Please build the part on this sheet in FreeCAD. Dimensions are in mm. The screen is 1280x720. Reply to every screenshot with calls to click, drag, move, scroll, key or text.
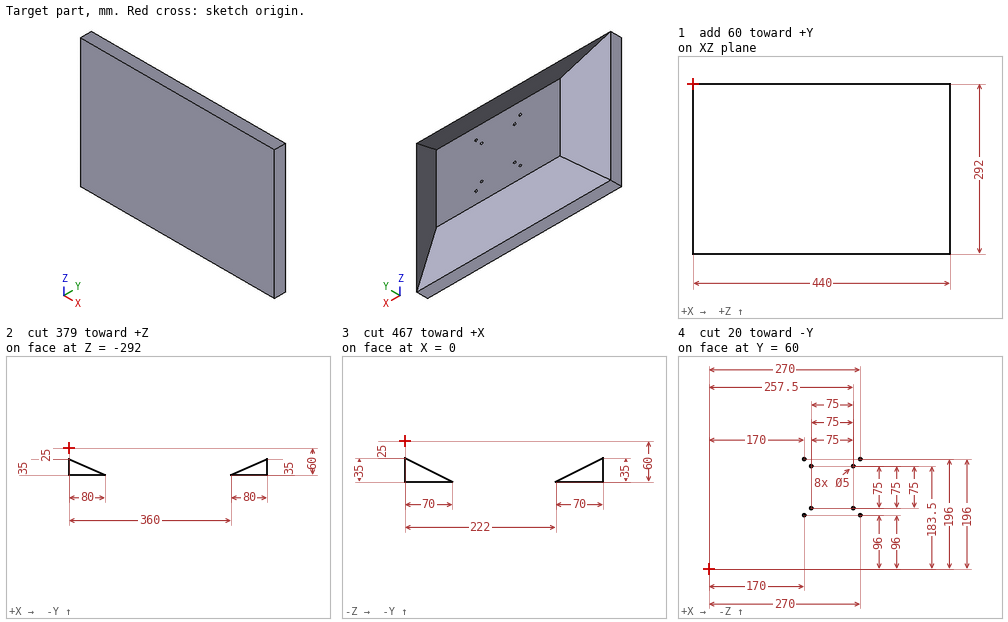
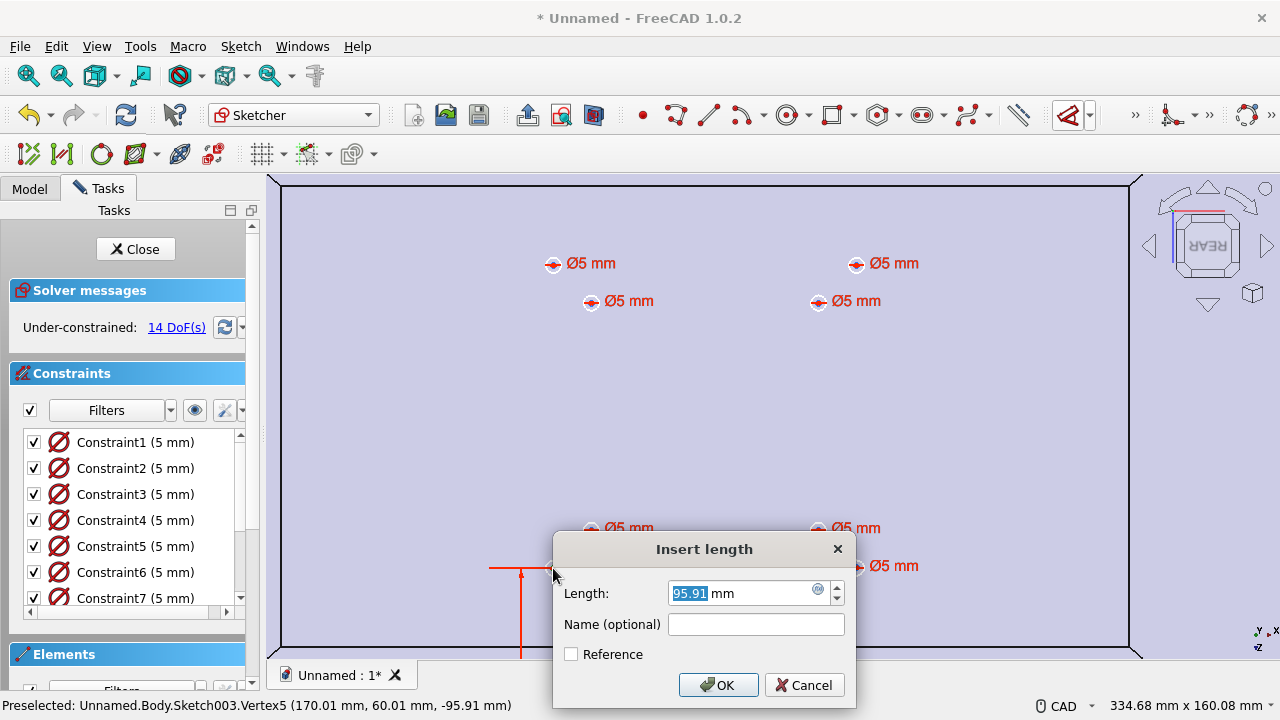
text(96)
key(Return)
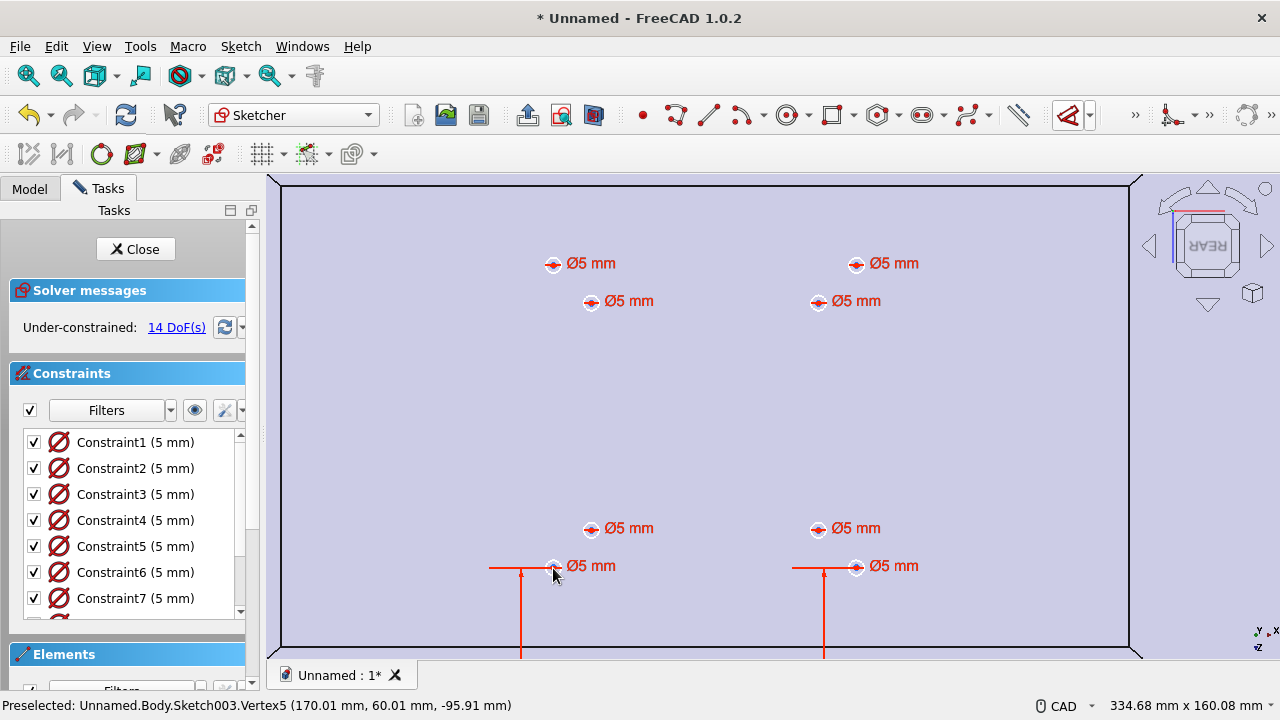
click(857, 265)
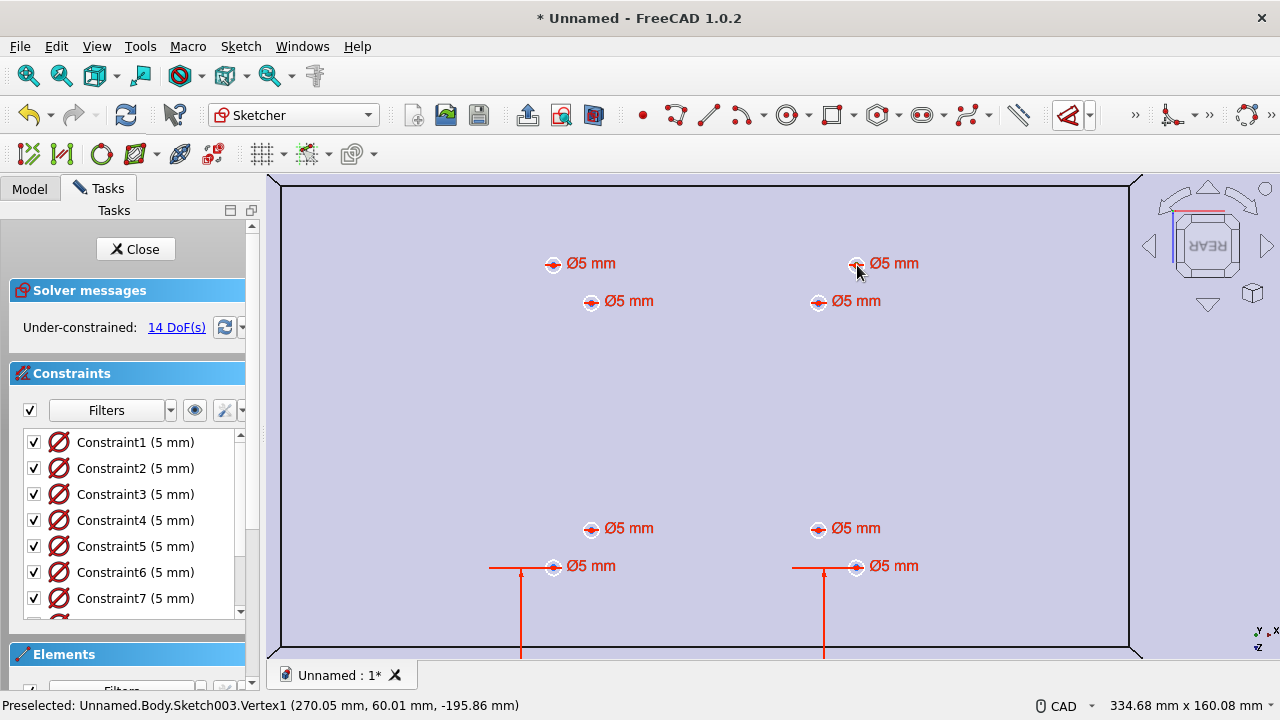
click(1090, 116)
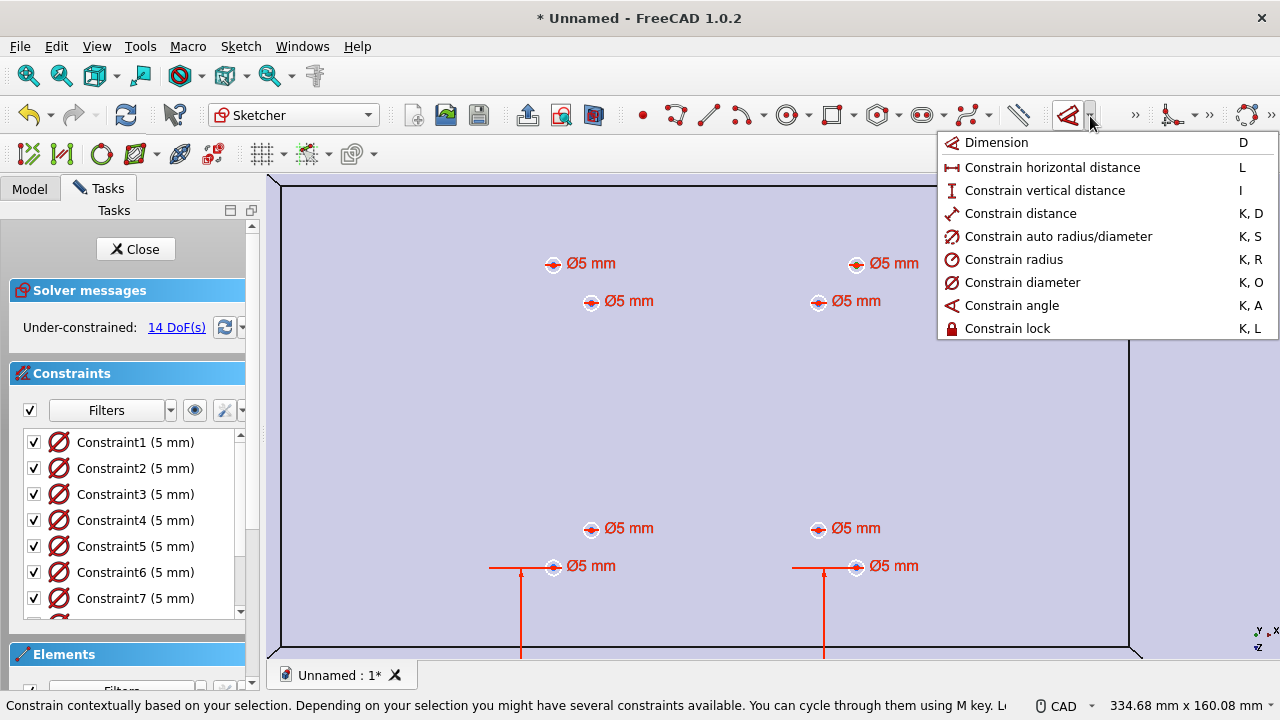
click(1108, 168)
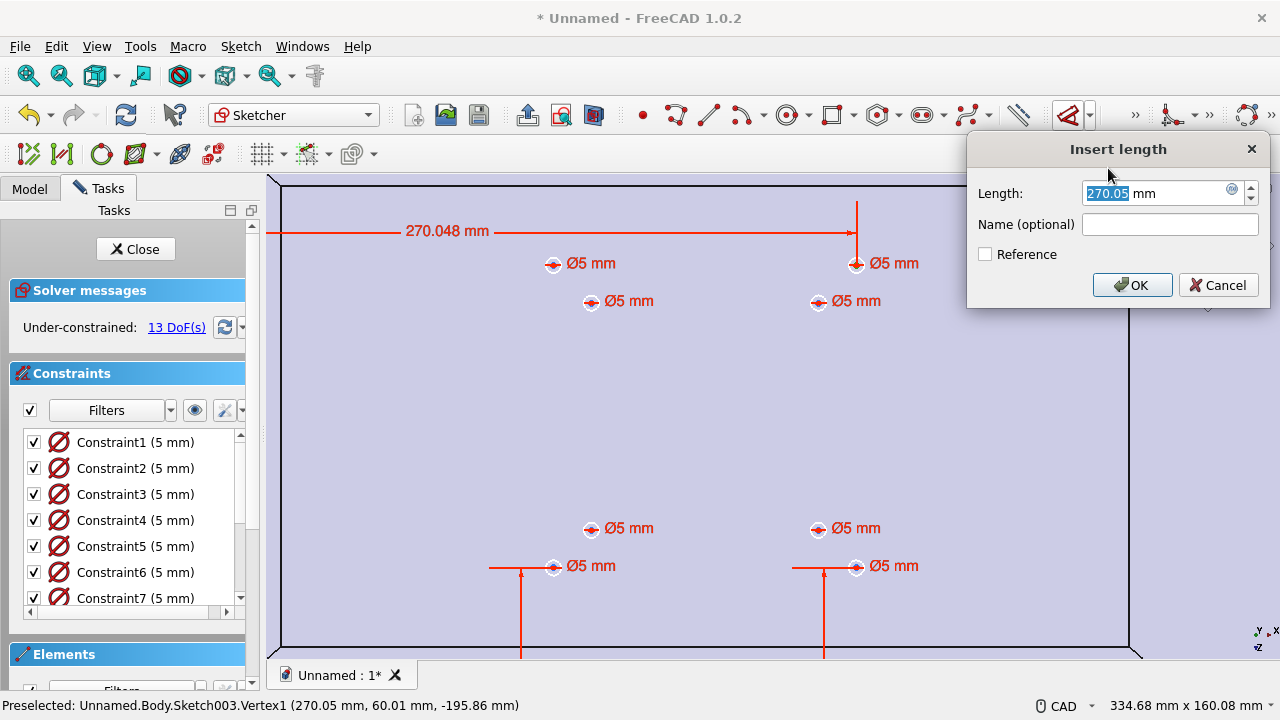
text(270)
key(Return)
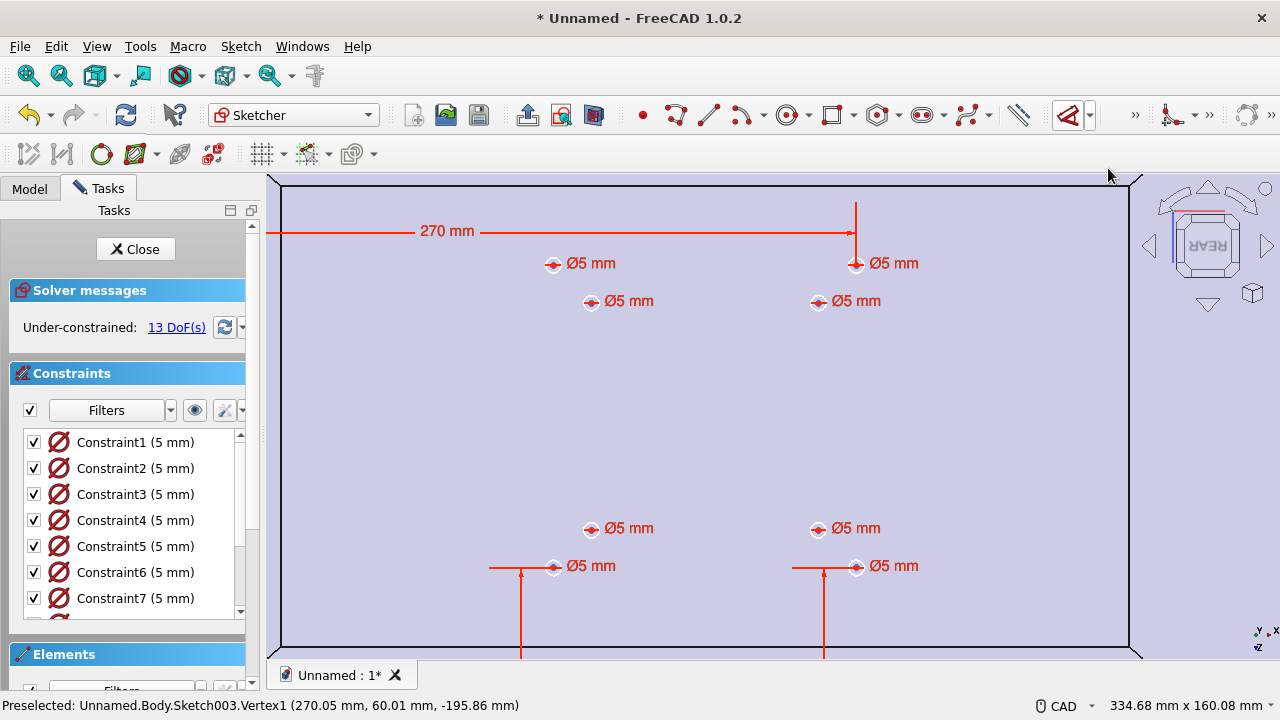
click(856, 265)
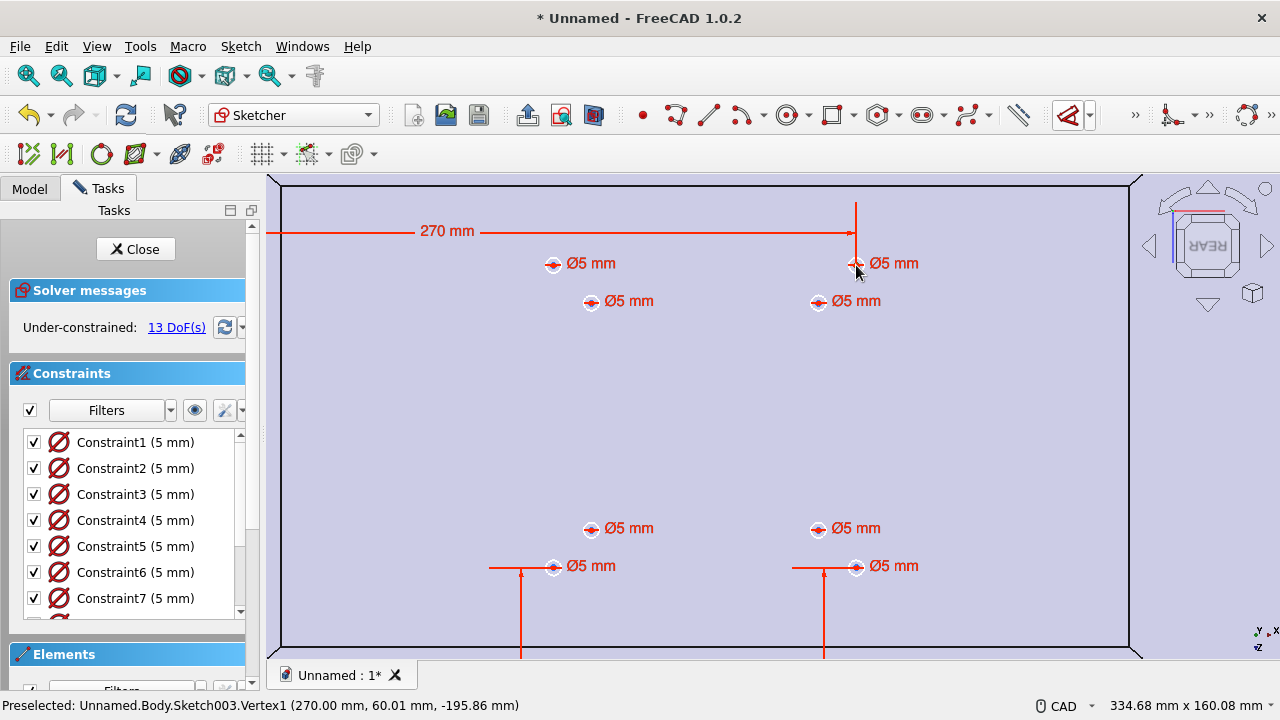
key(i)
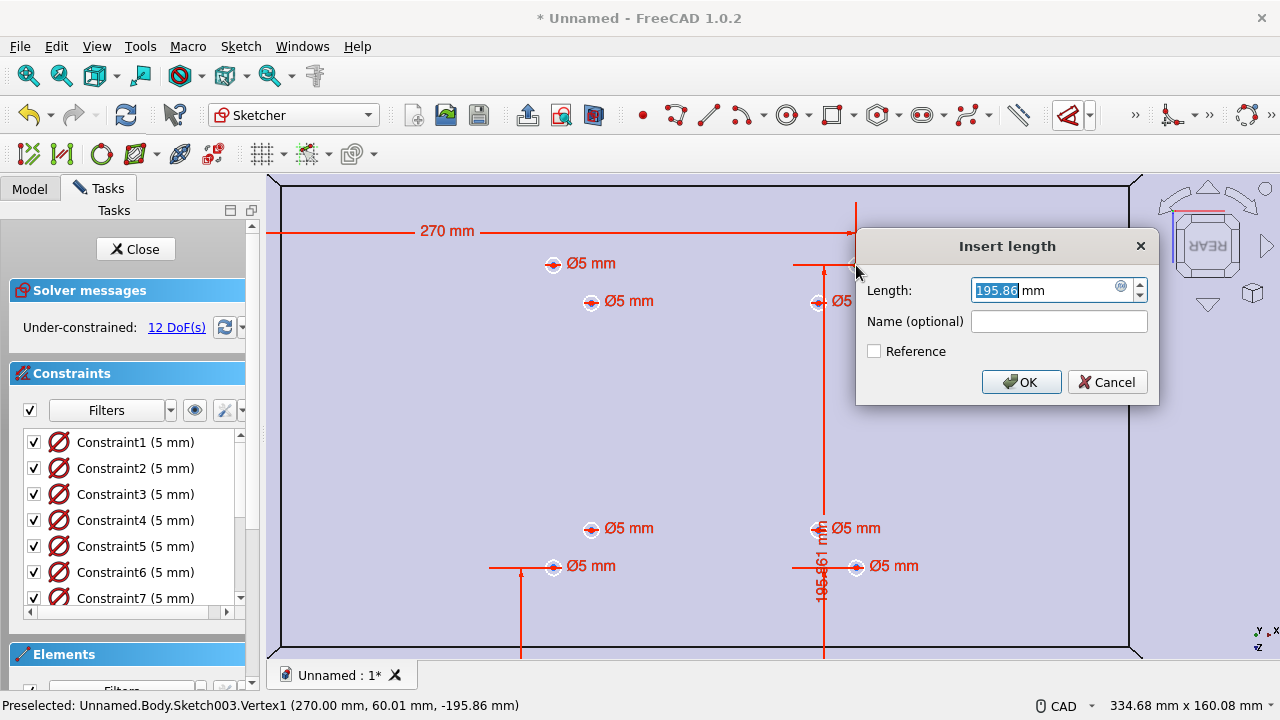
text(196)
key(Return)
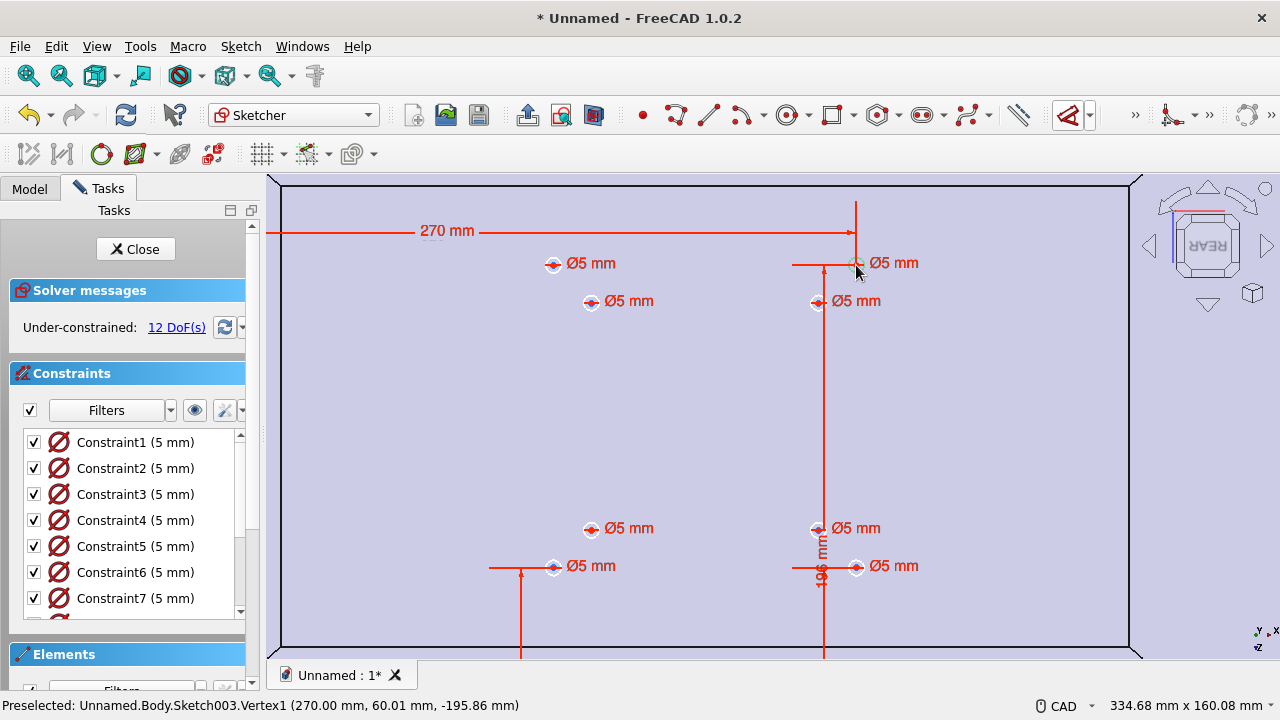
click(856, 568)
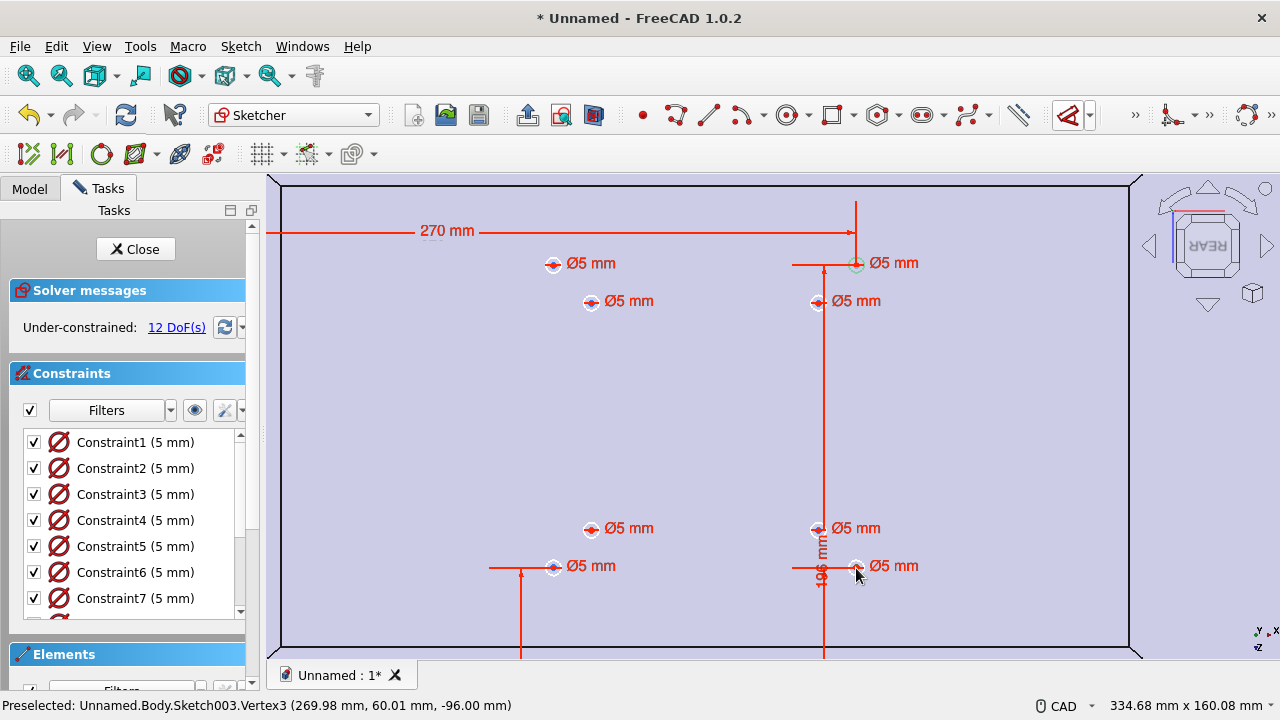
click(1090, 116)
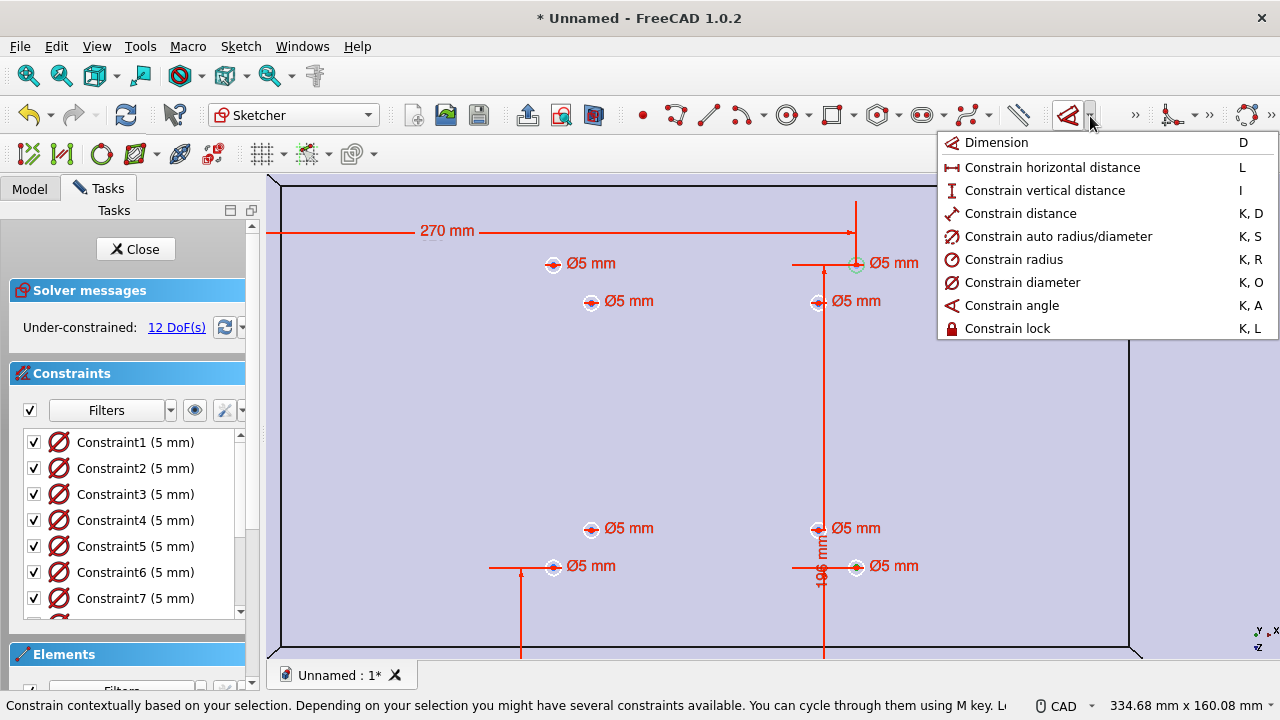
click(1108, 168)